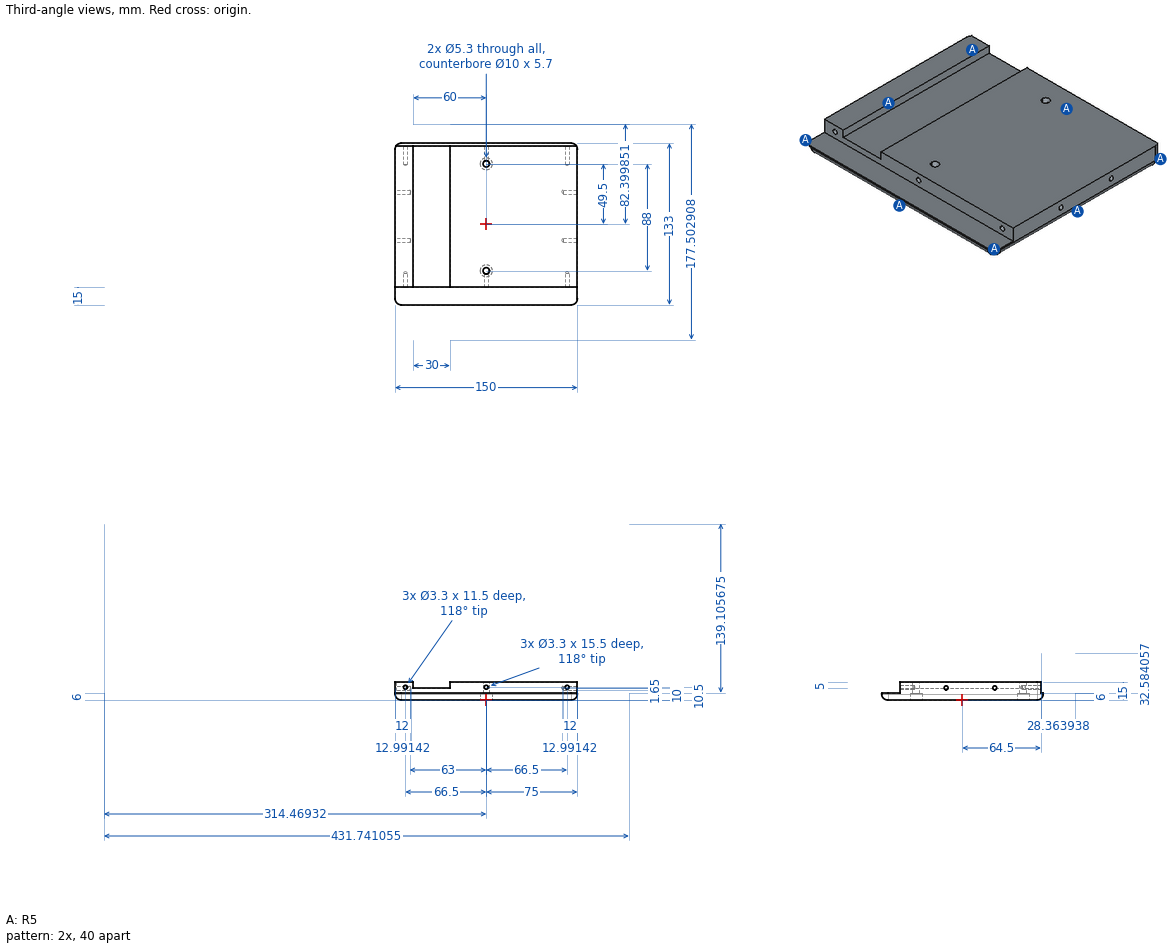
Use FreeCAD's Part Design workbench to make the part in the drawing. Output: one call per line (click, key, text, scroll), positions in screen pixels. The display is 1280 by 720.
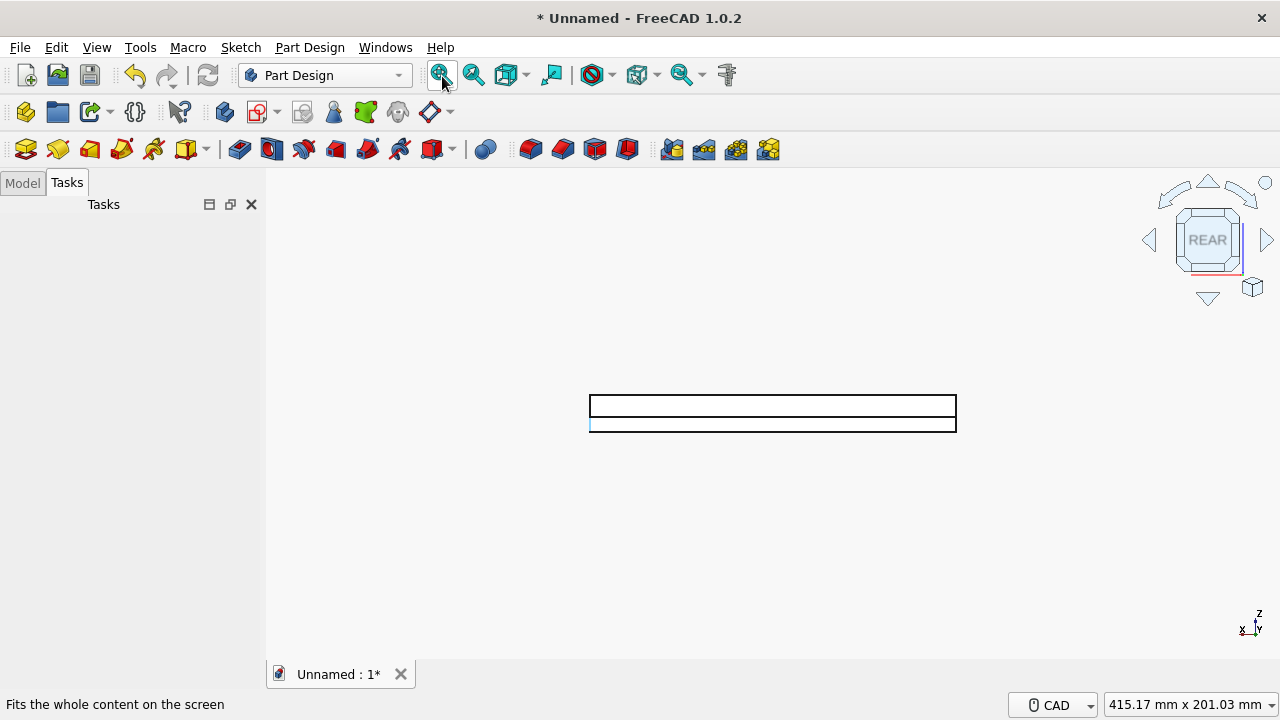
click(956, 423, ctrl)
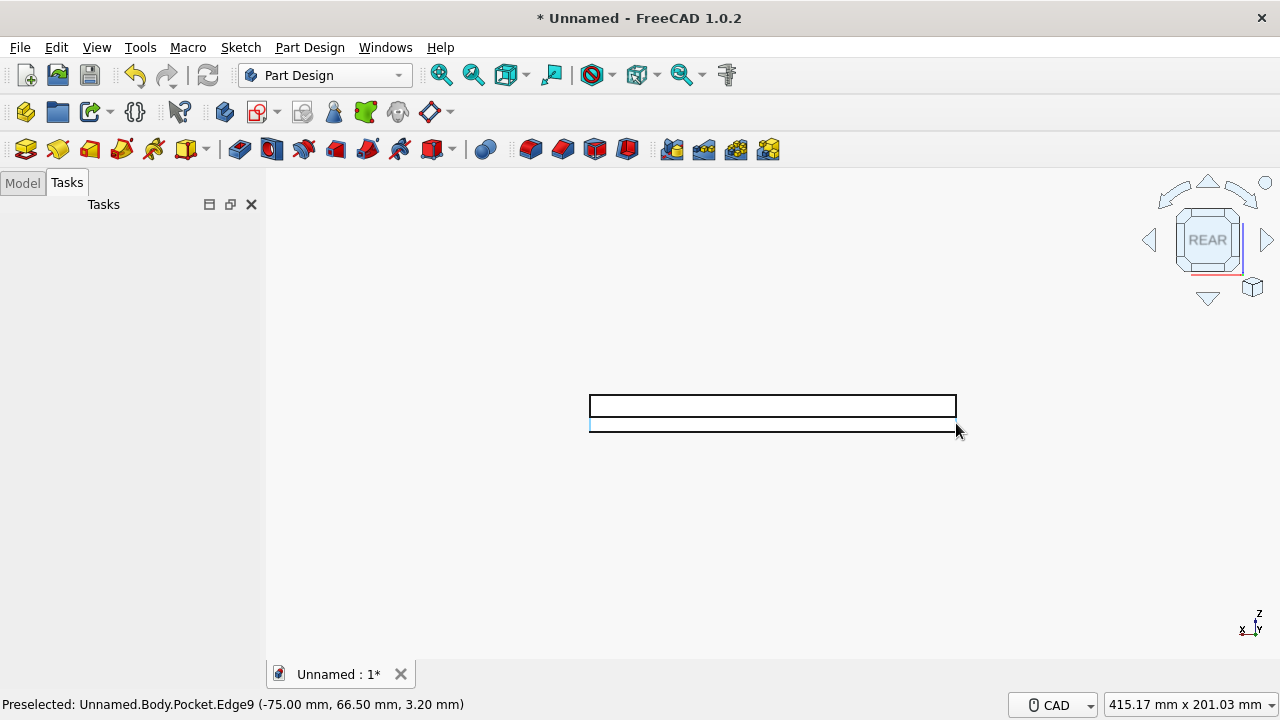
click(532, 150)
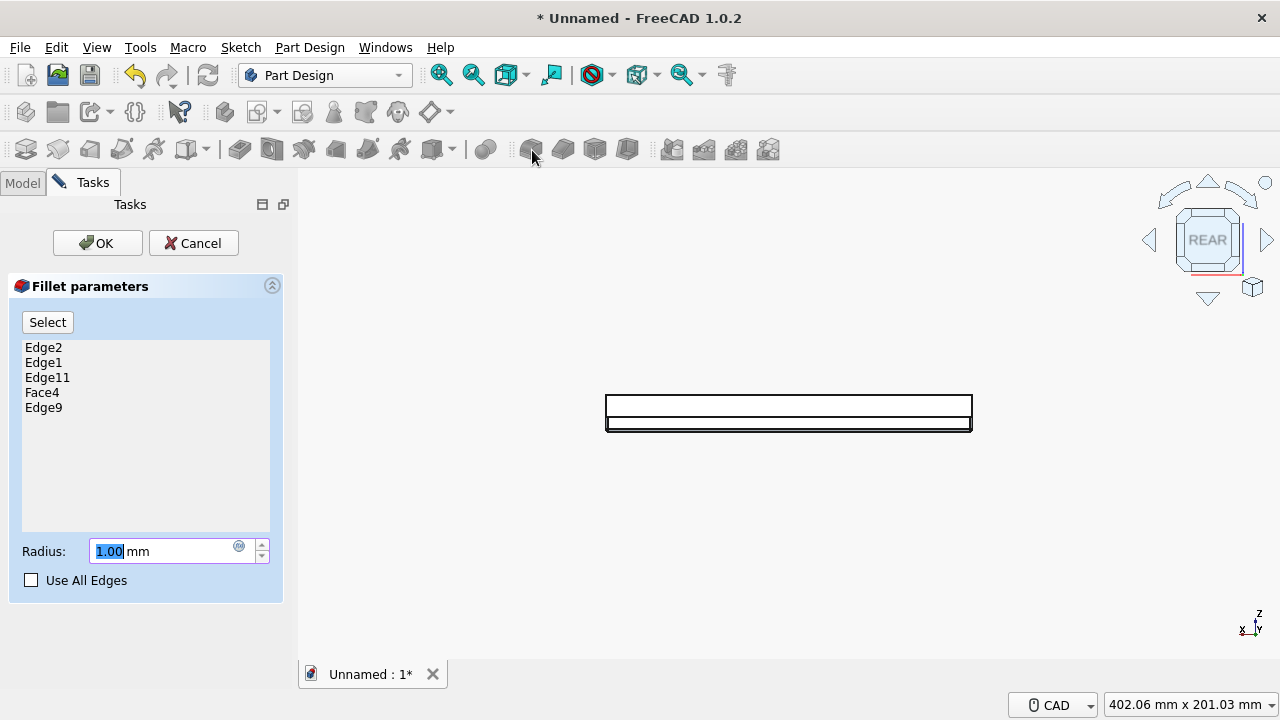
text(5)
key(Tab)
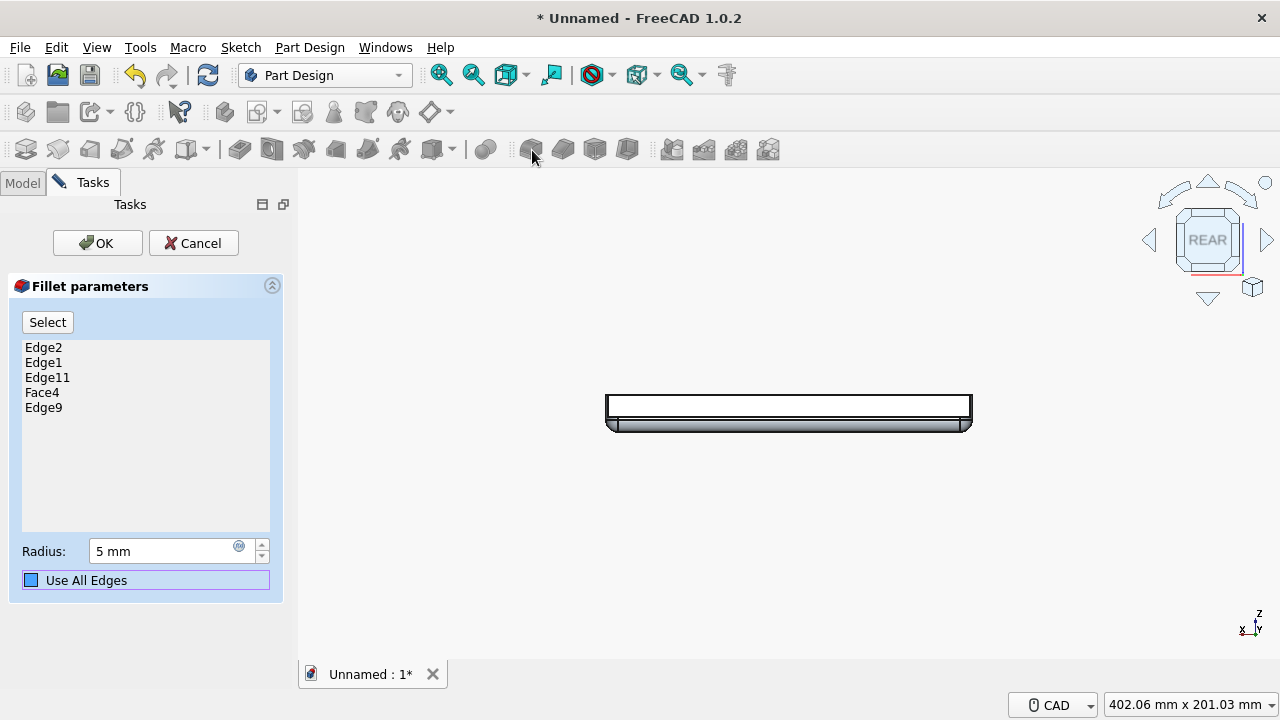
click(98, 243)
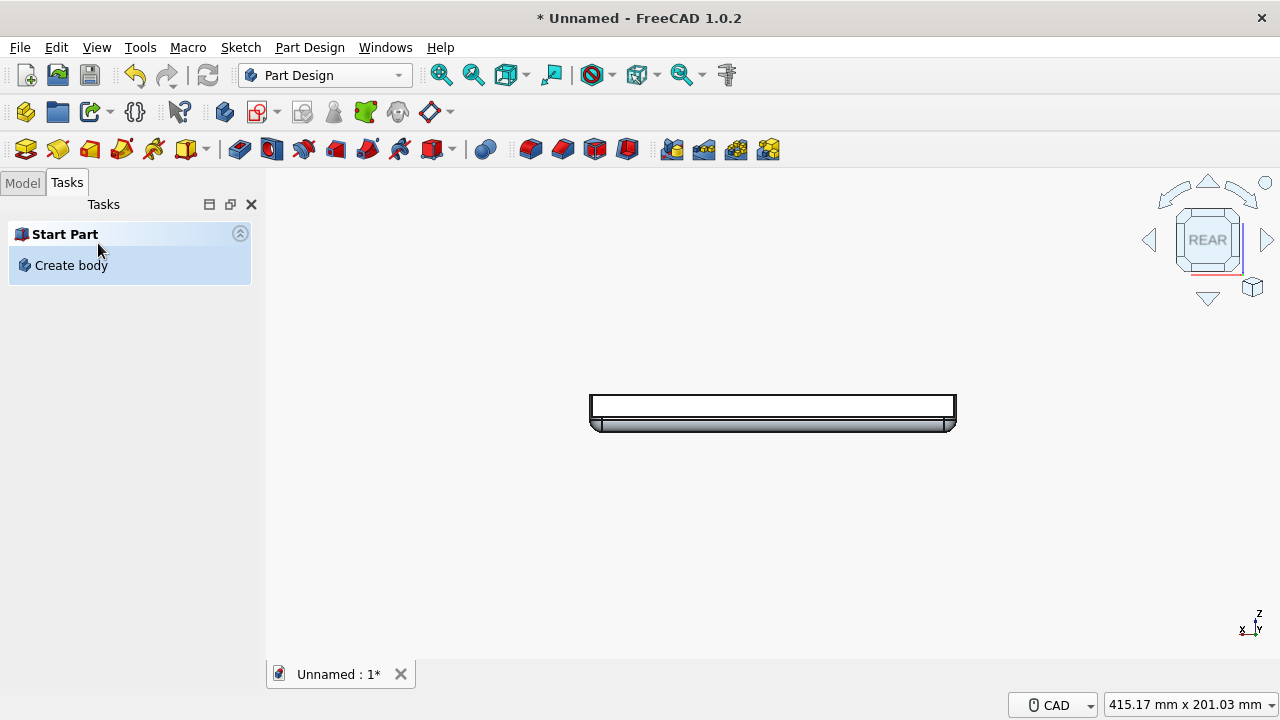
click(442, 76)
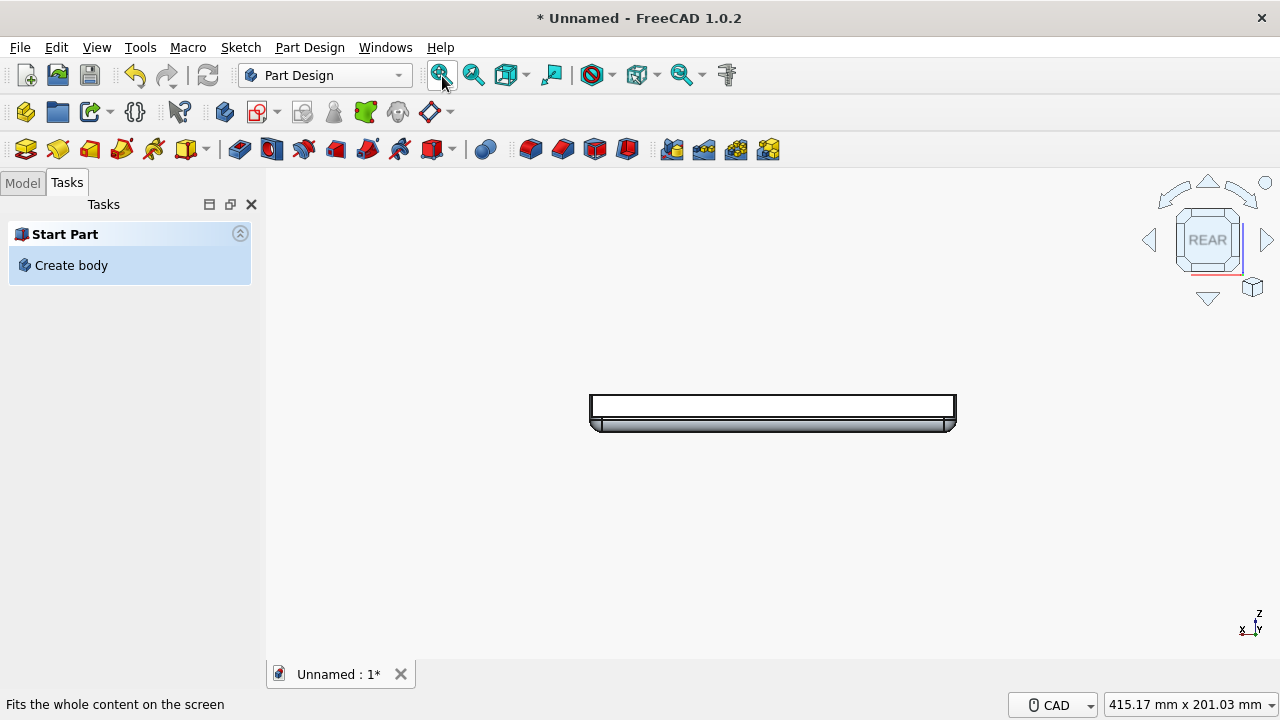
key(5)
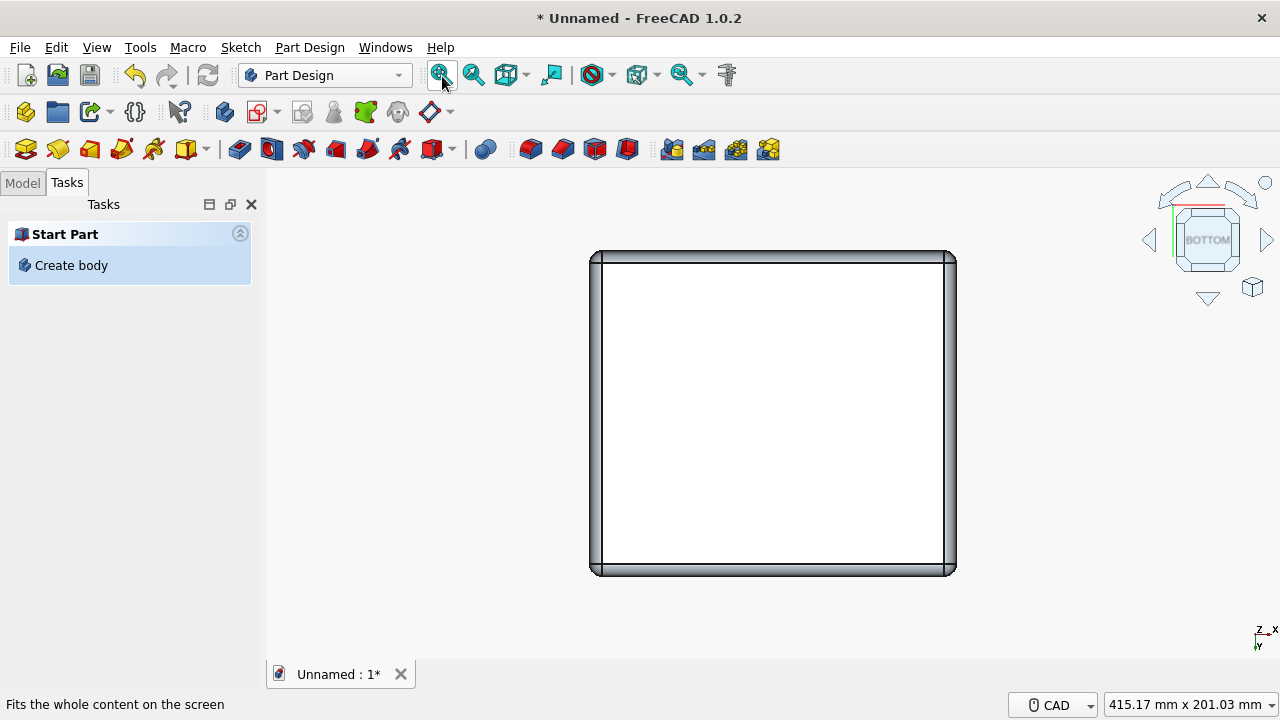
click(773, 412)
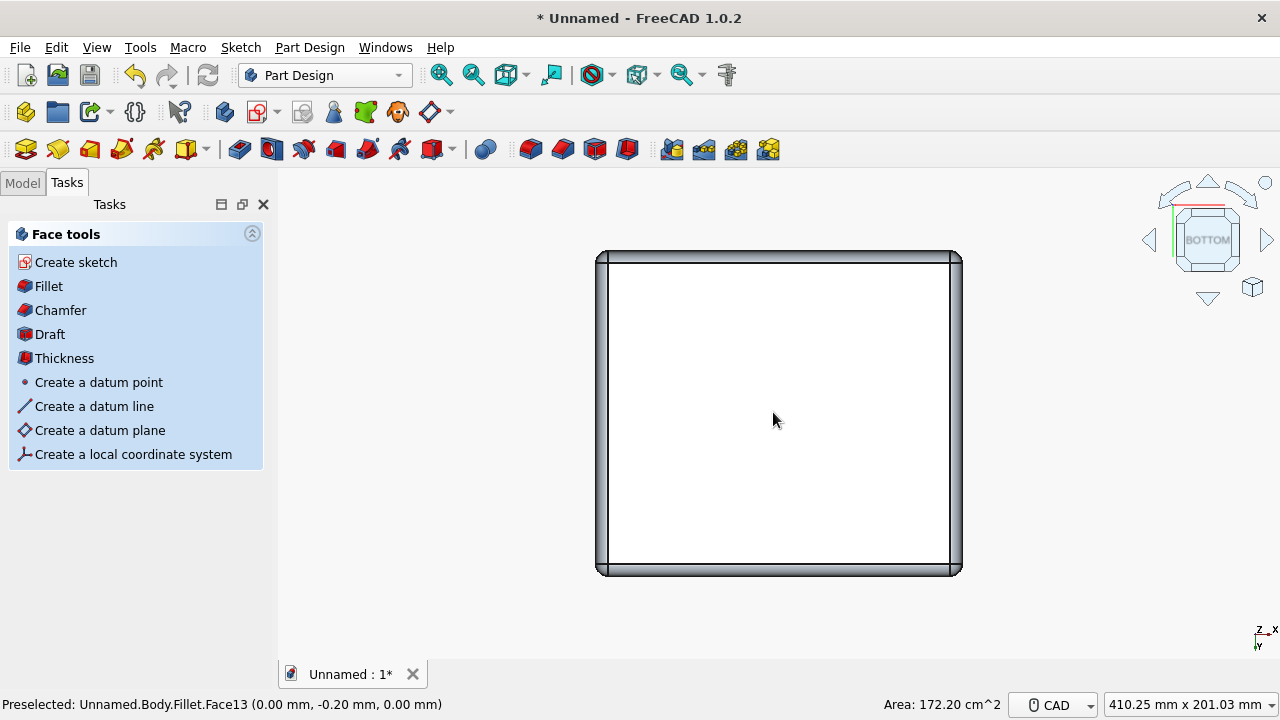
click(258, 112)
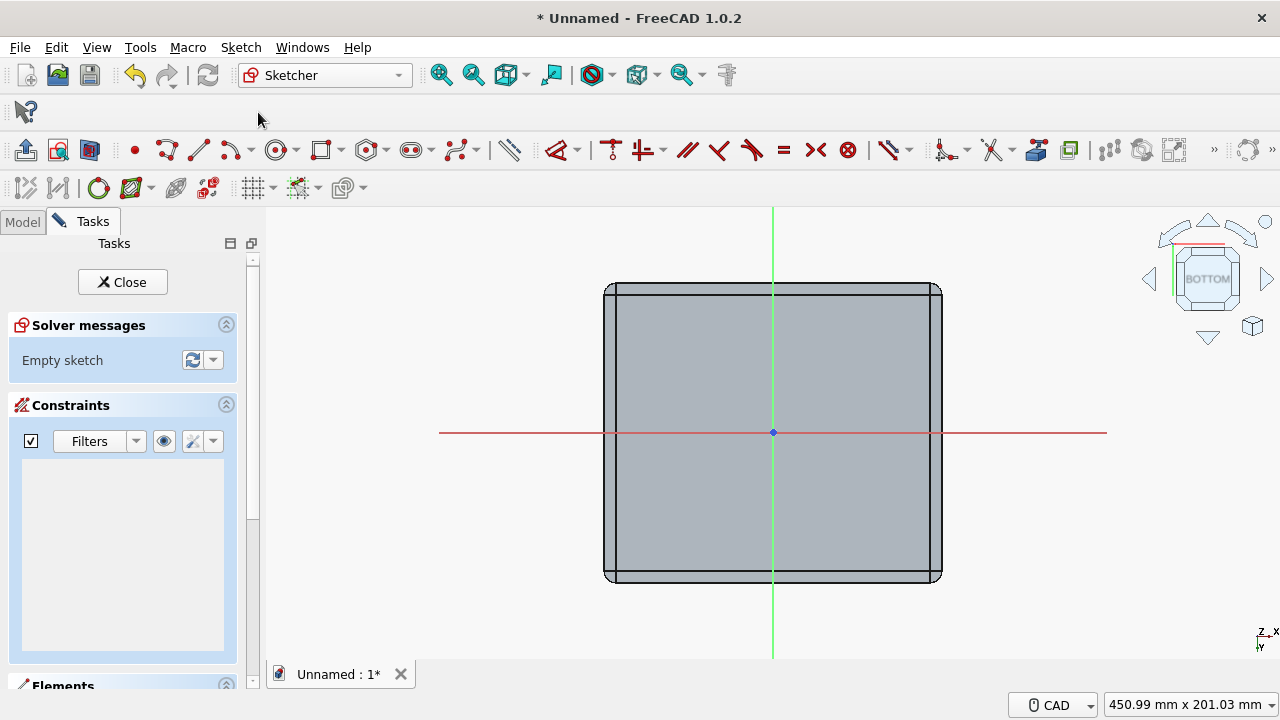
click(276, 150)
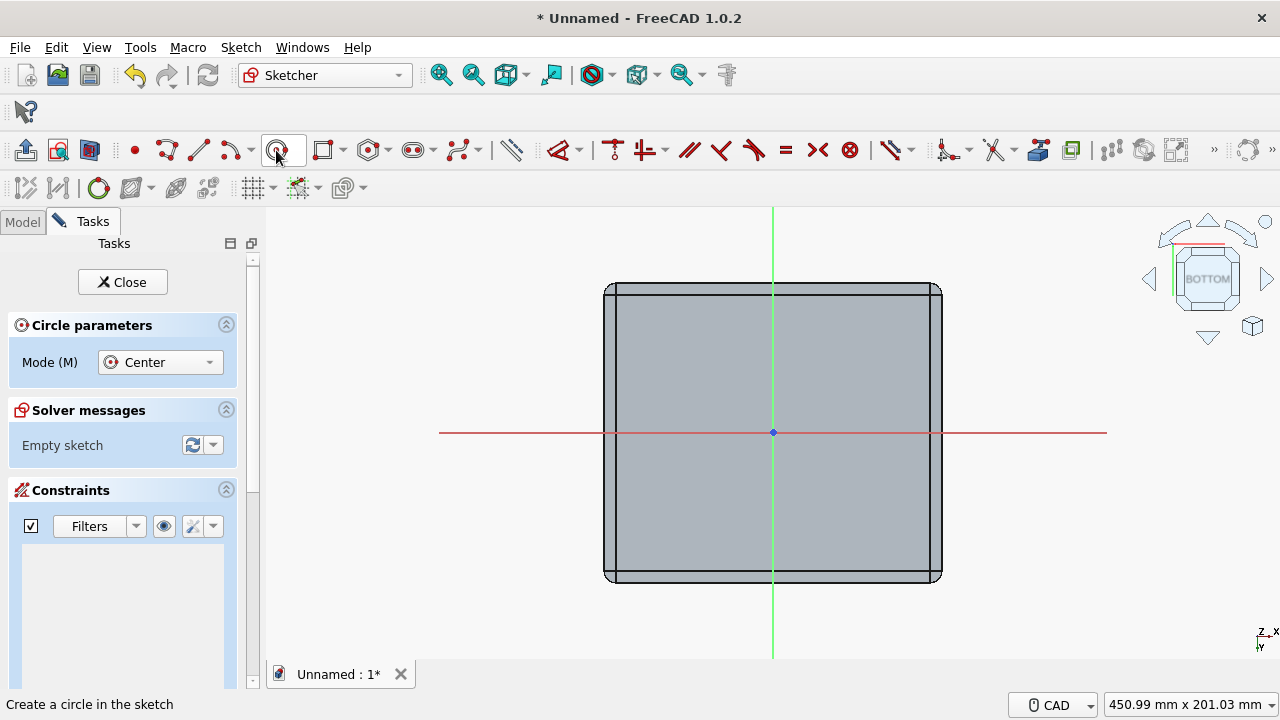
scroll(773, 544, up, 7)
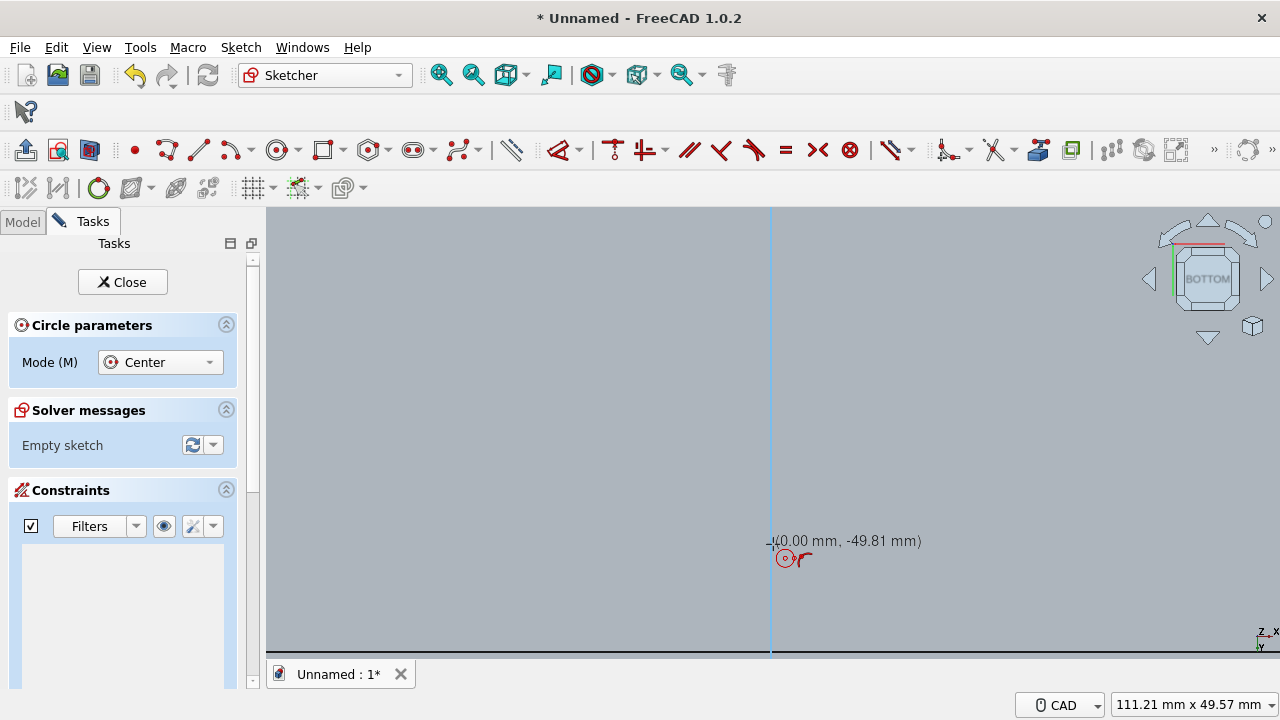
scroll(676, 559, down, 6)